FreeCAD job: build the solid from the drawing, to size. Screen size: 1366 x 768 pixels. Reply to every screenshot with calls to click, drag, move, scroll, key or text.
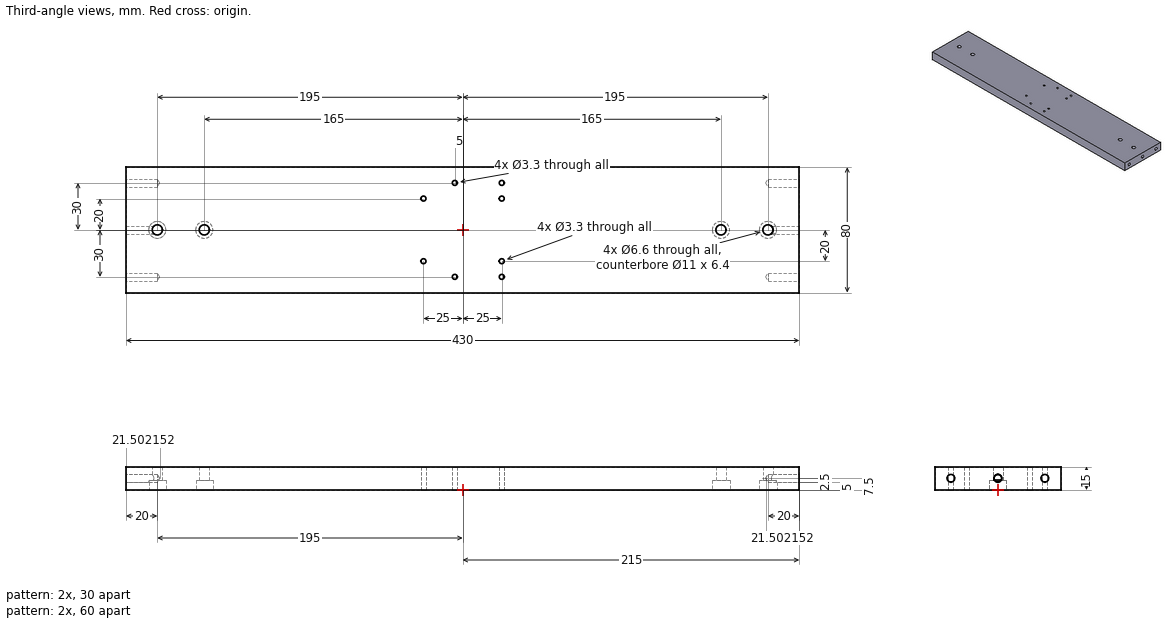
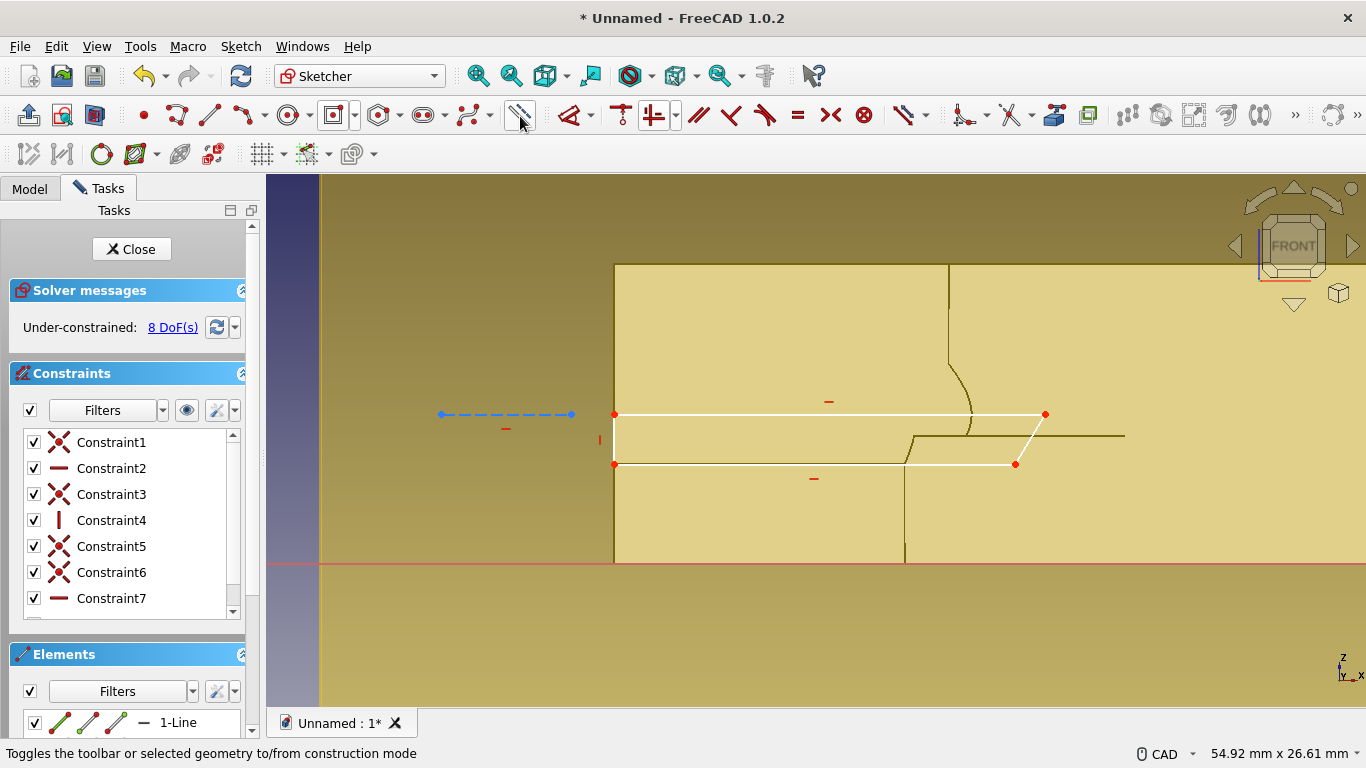
click(568, 116)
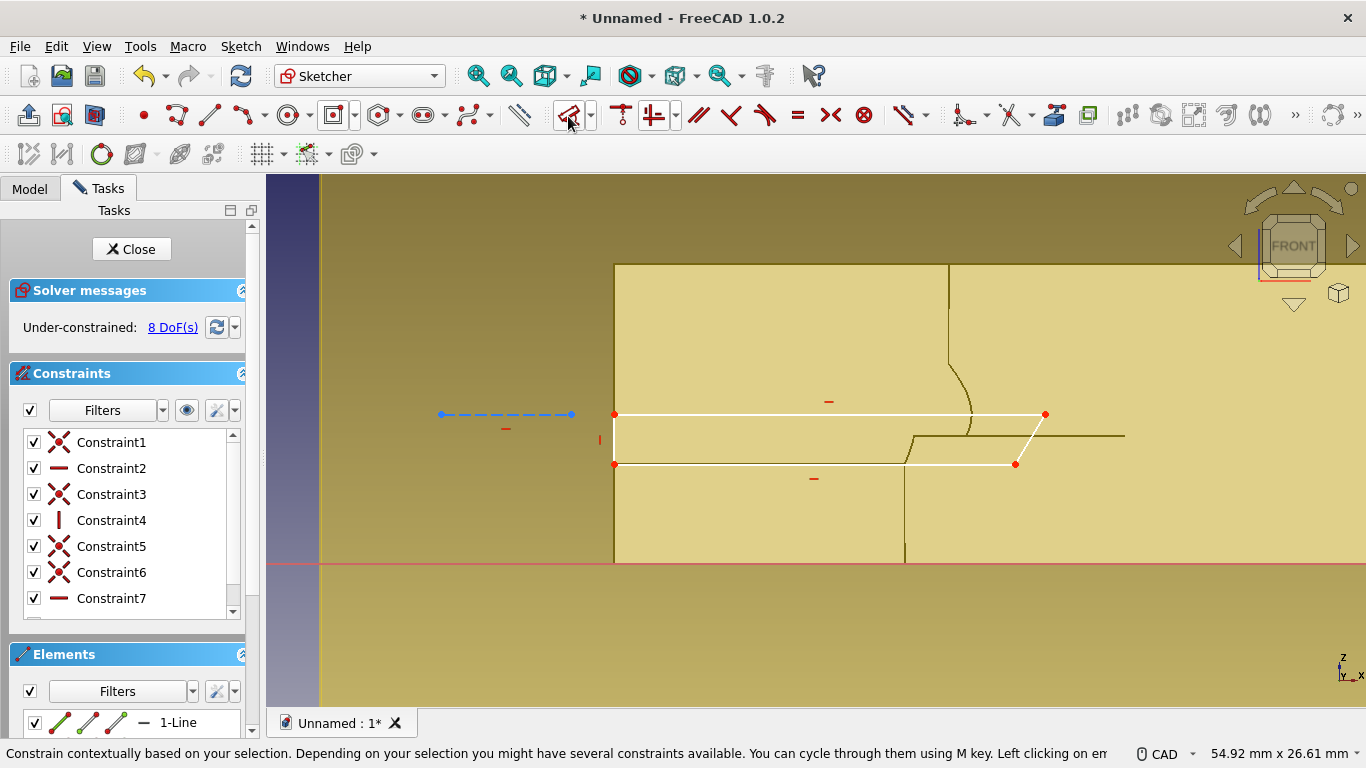
click(895, 465)
click(815, 499)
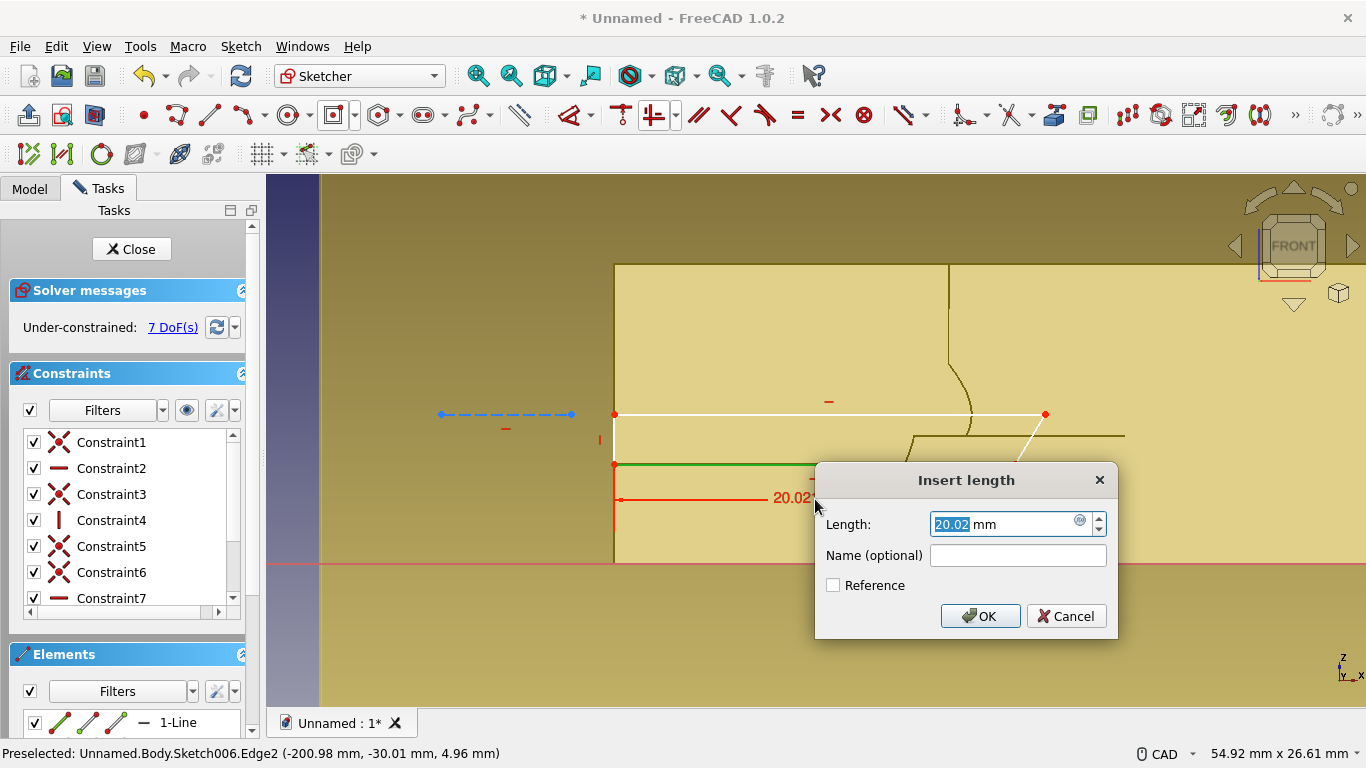
text(20)
key(Return)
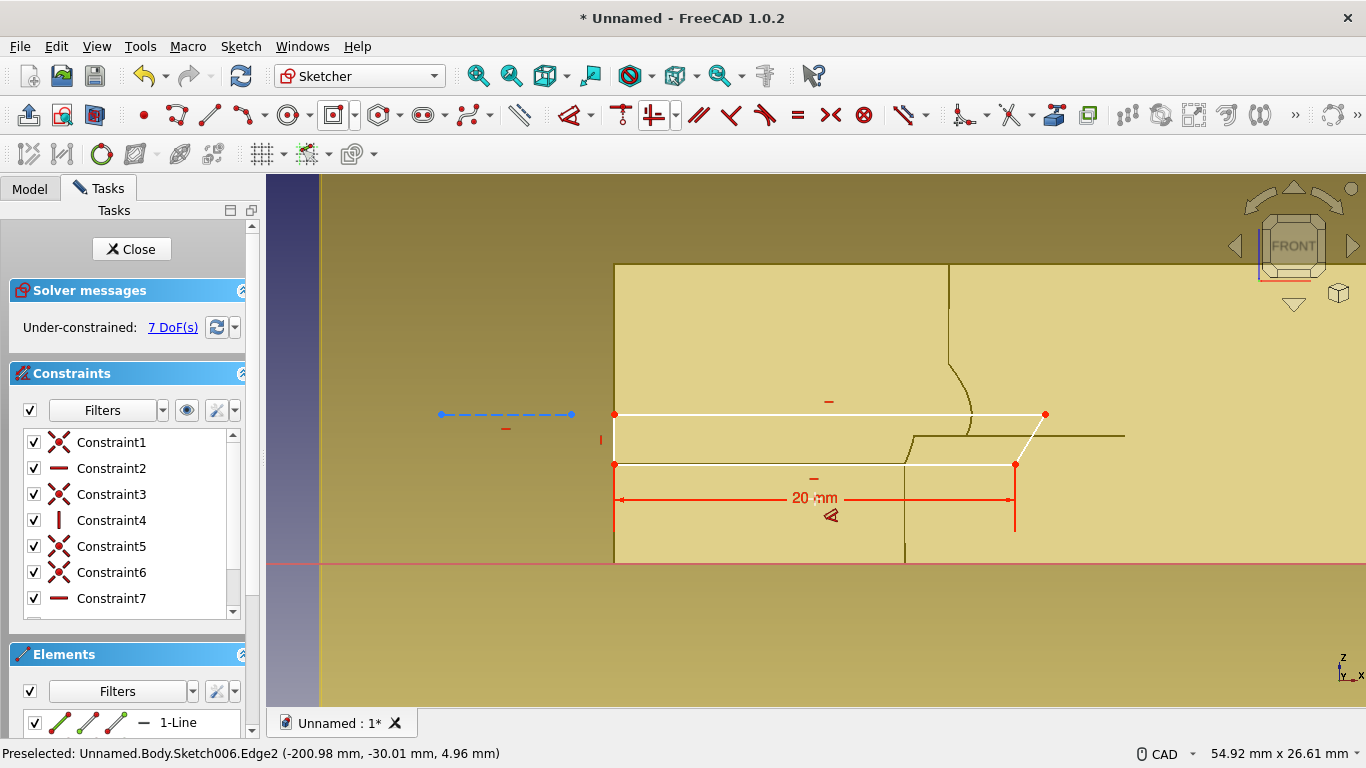
click(1015, 465)
click(981, 515)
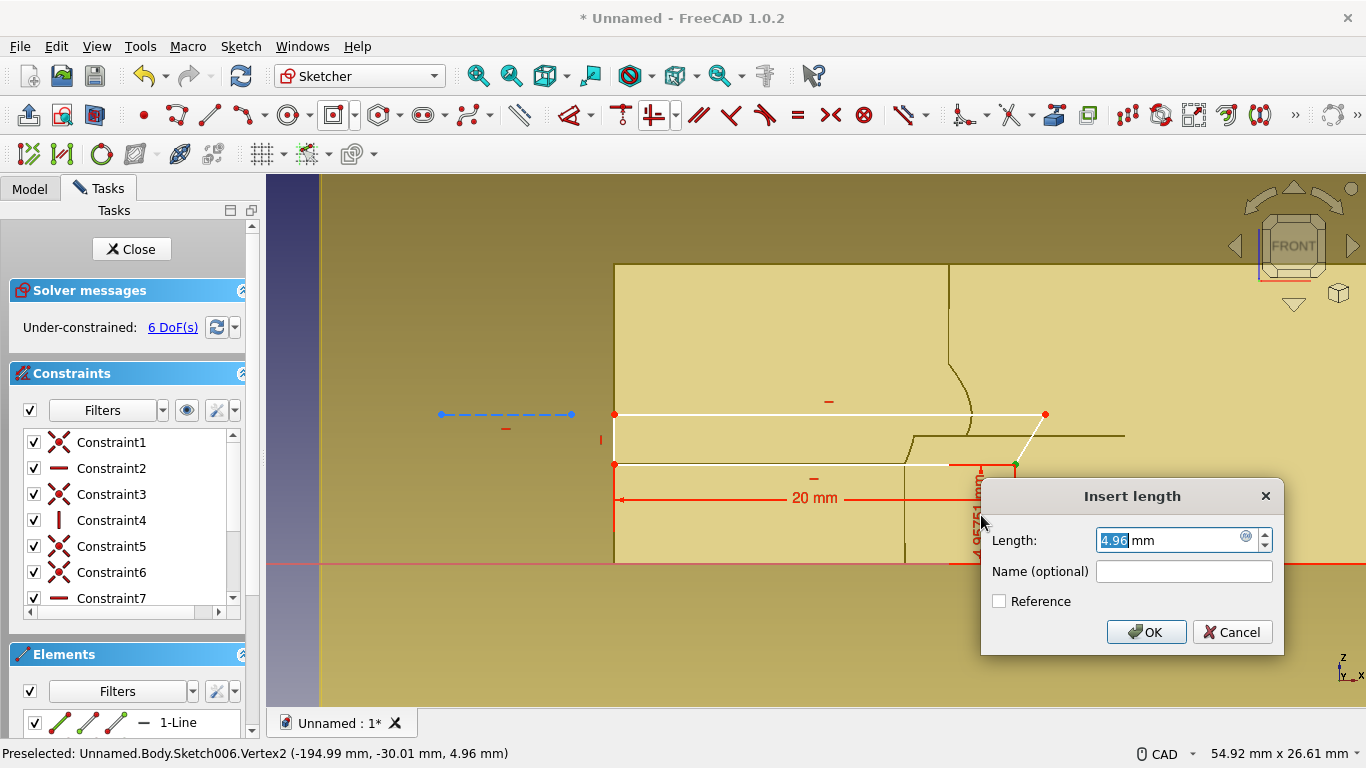
text(5)
key(Return)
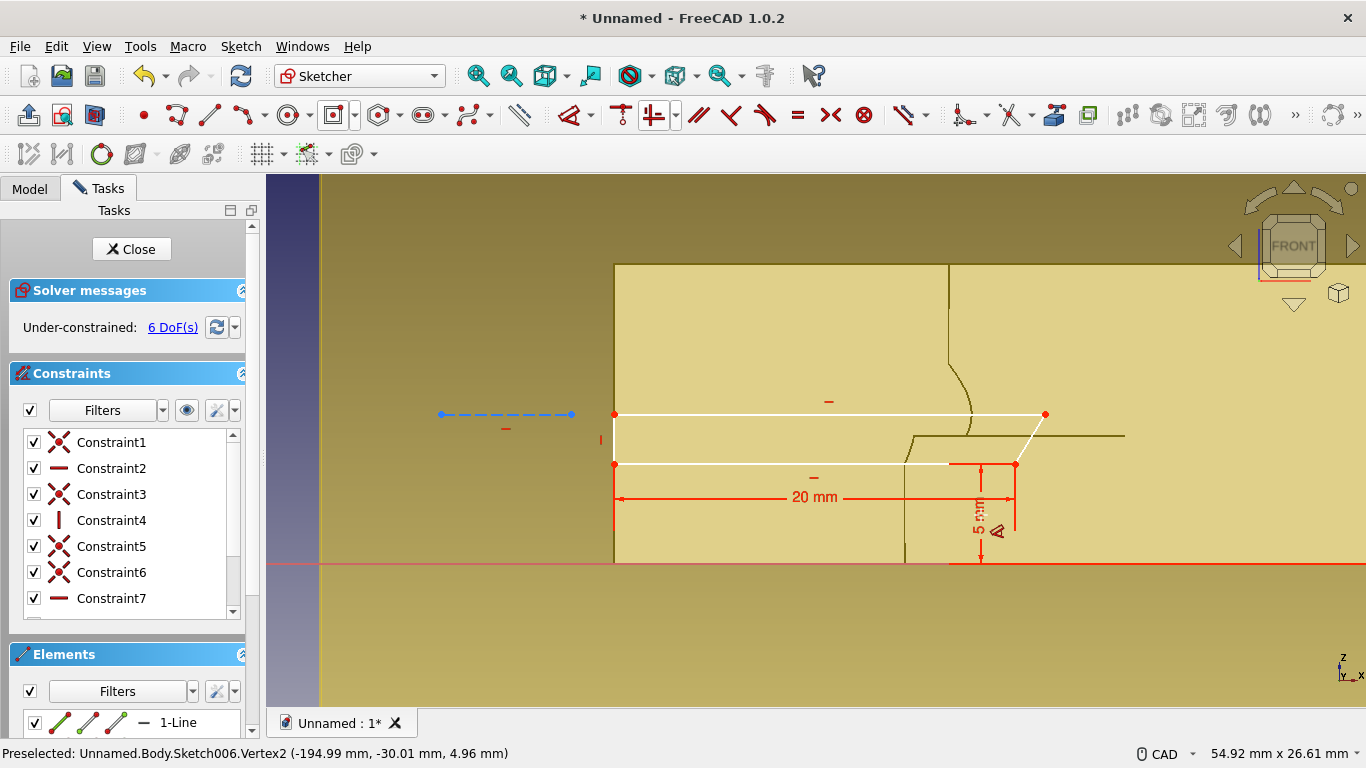
click(614, 449)
click(580, 440)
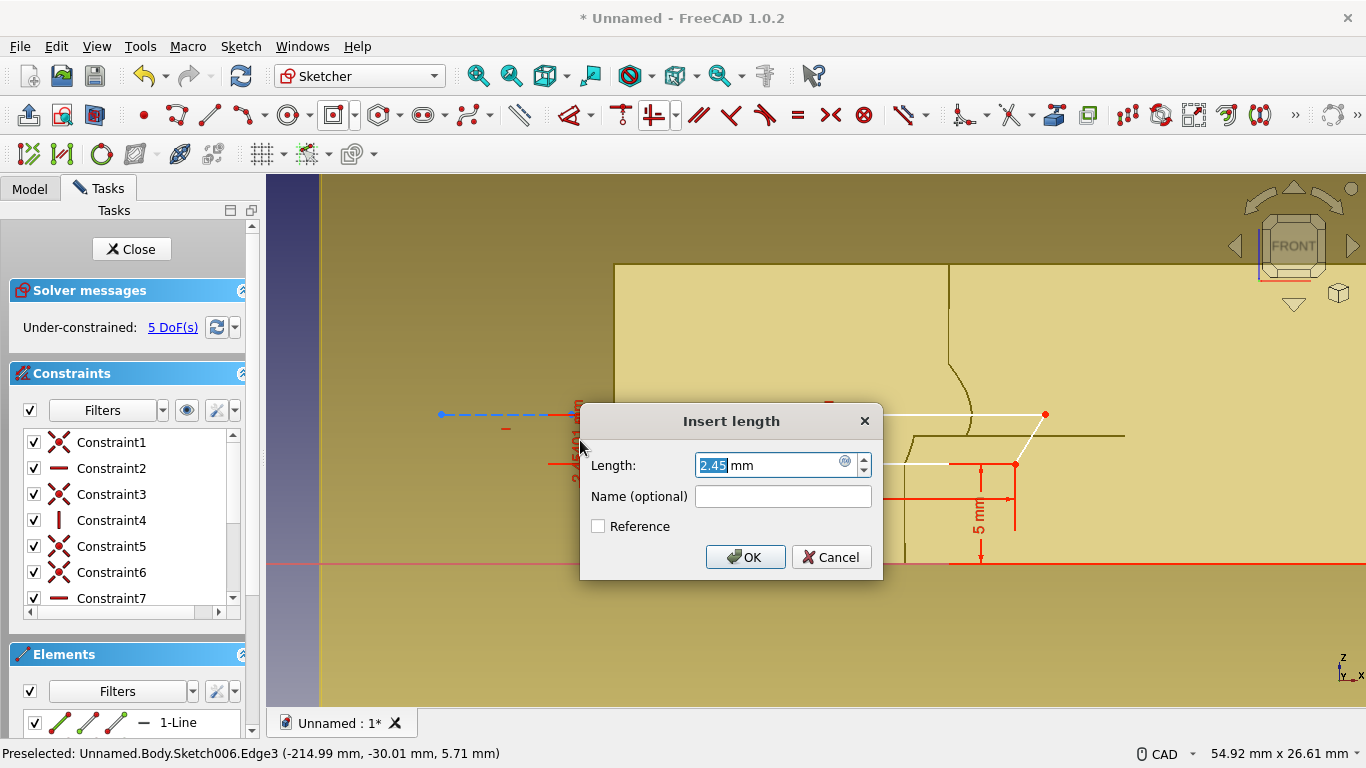
text(2.5)
key(Return)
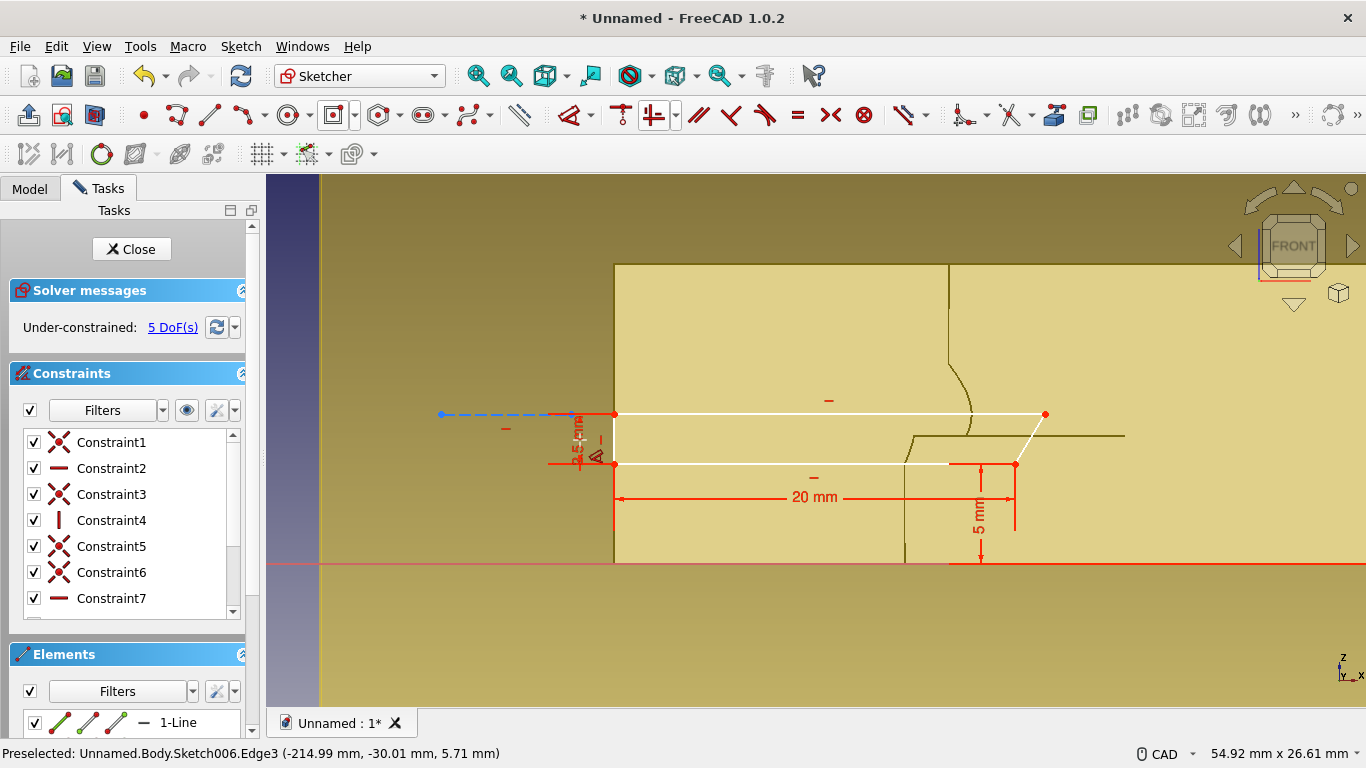
click(1015, 464)
click(1108, 598)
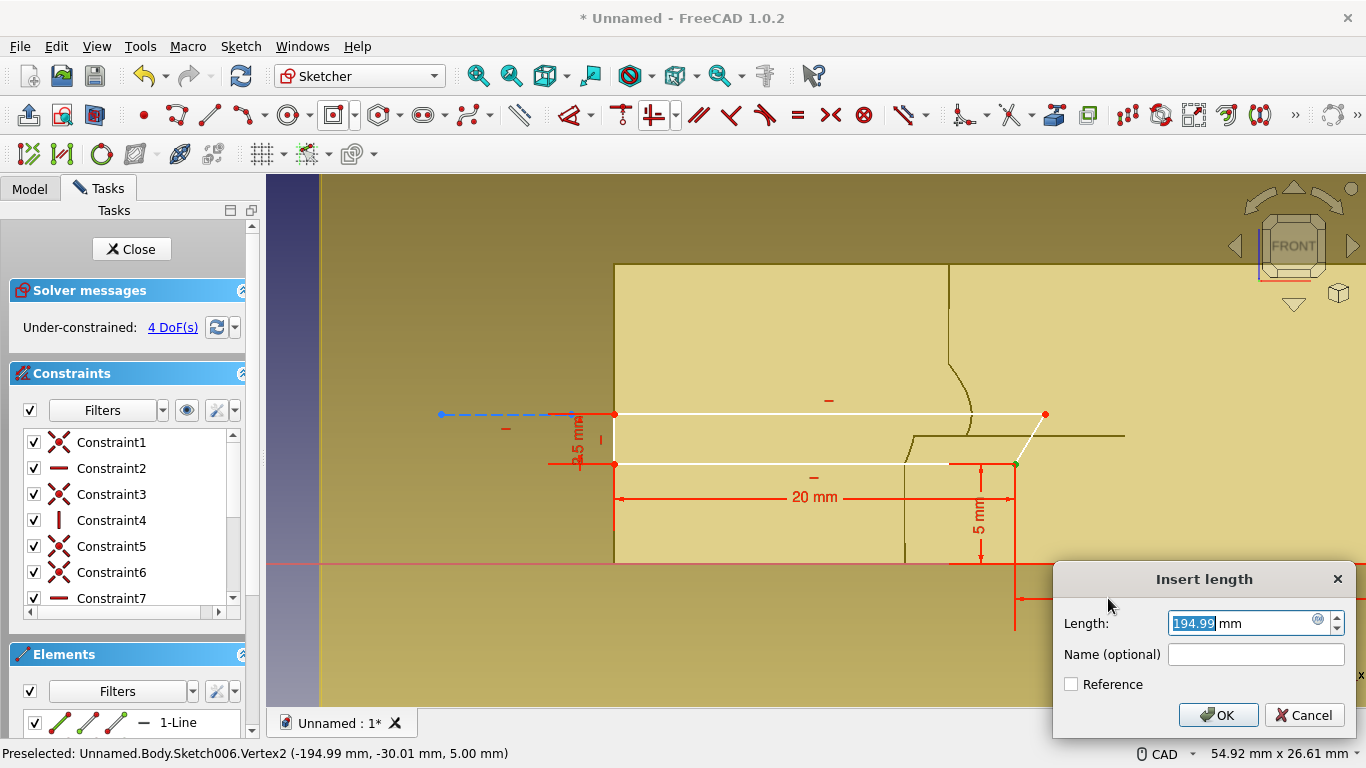
text(195)
key(Return)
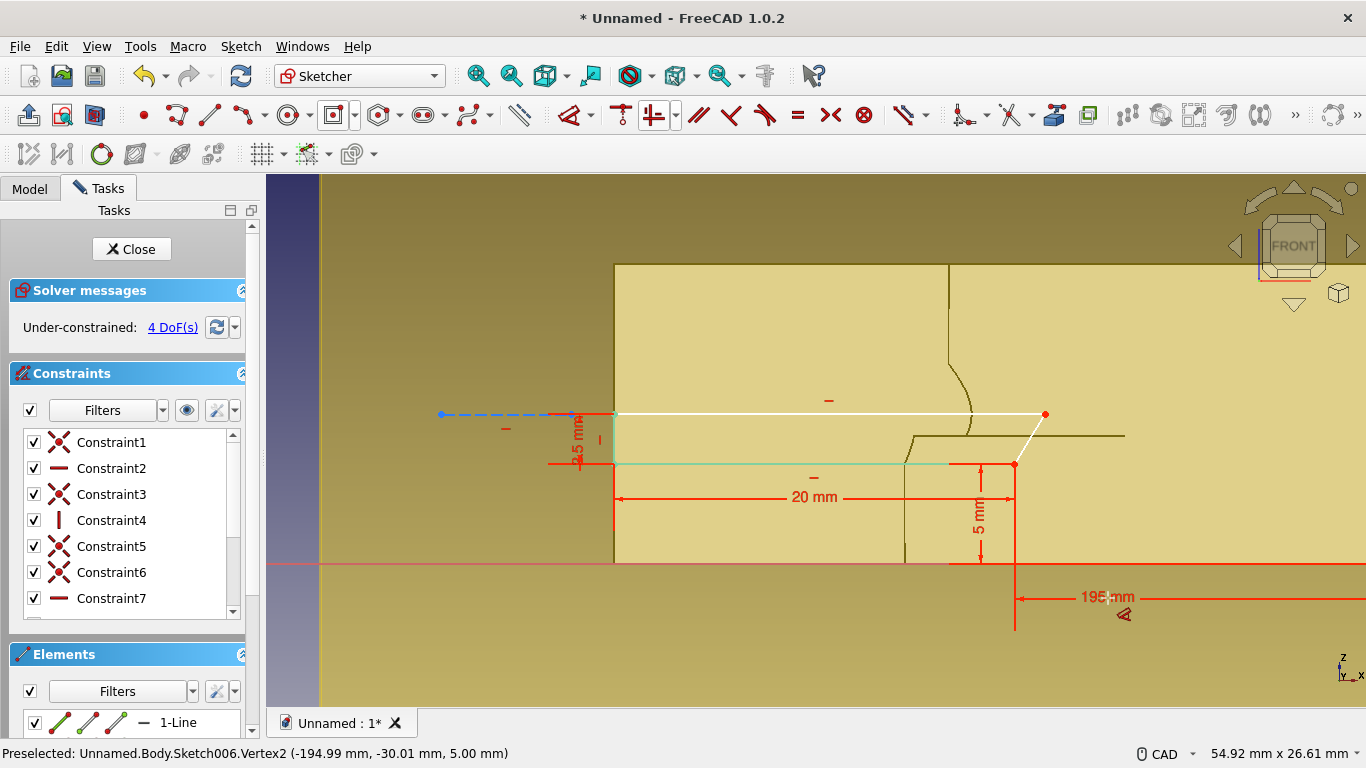
click(571, 415)
click(537, 490)